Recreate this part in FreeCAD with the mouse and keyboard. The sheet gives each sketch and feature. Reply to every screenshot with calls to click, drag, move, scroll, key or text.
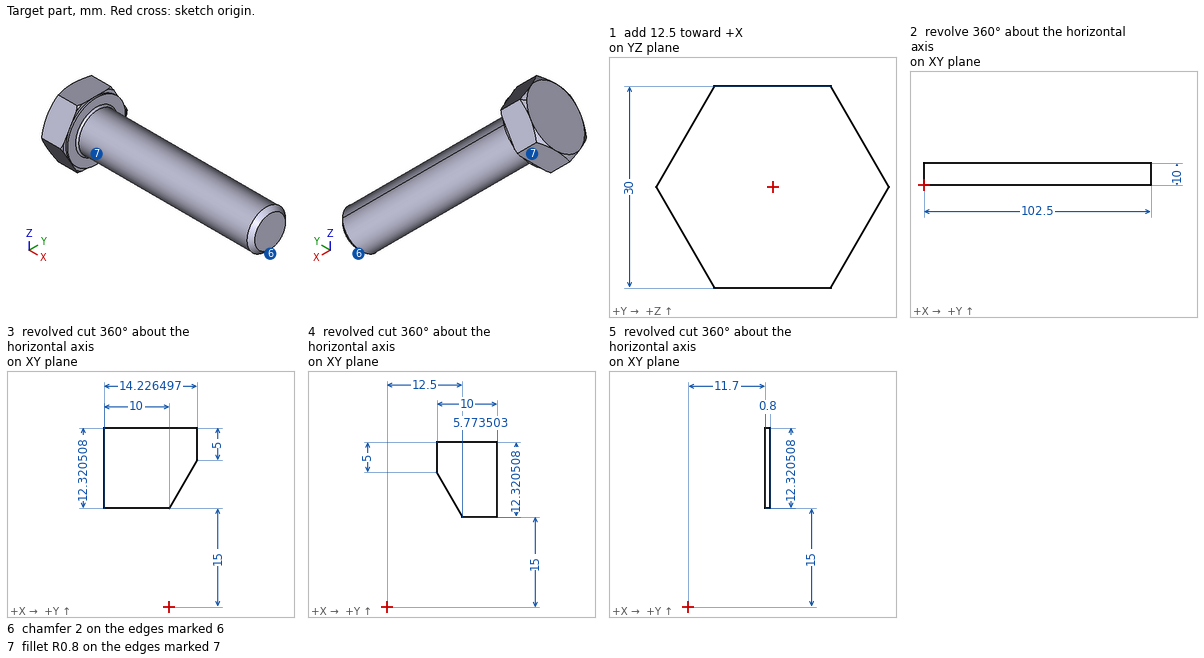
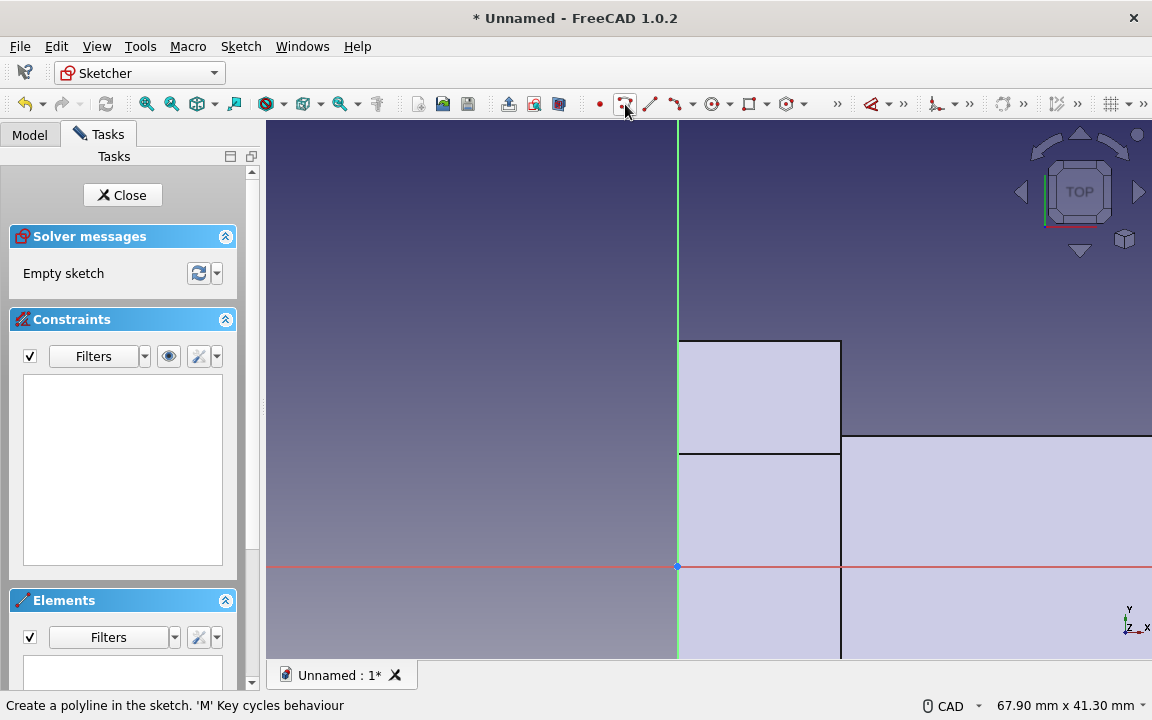
click(678, 371)
click(733, 276)
click(733, 210)
click(547, 210)
click(547, 371)
click(678, 372)
key(Escape)
key(Escape)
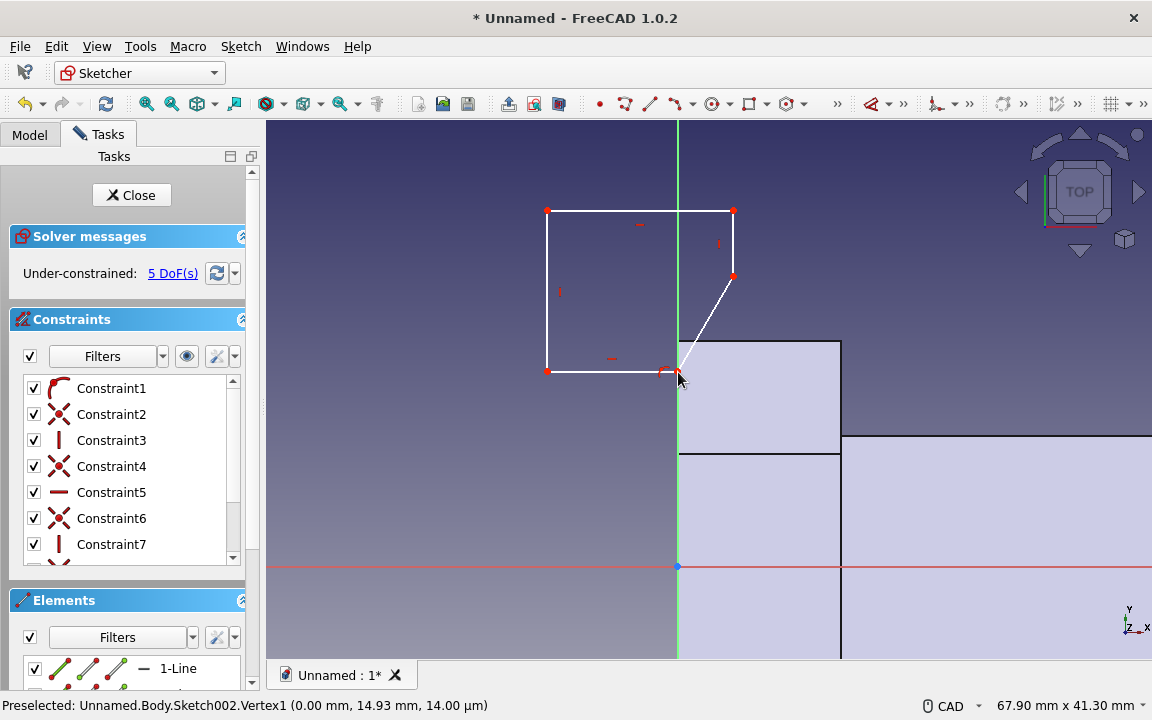
click(733, 257)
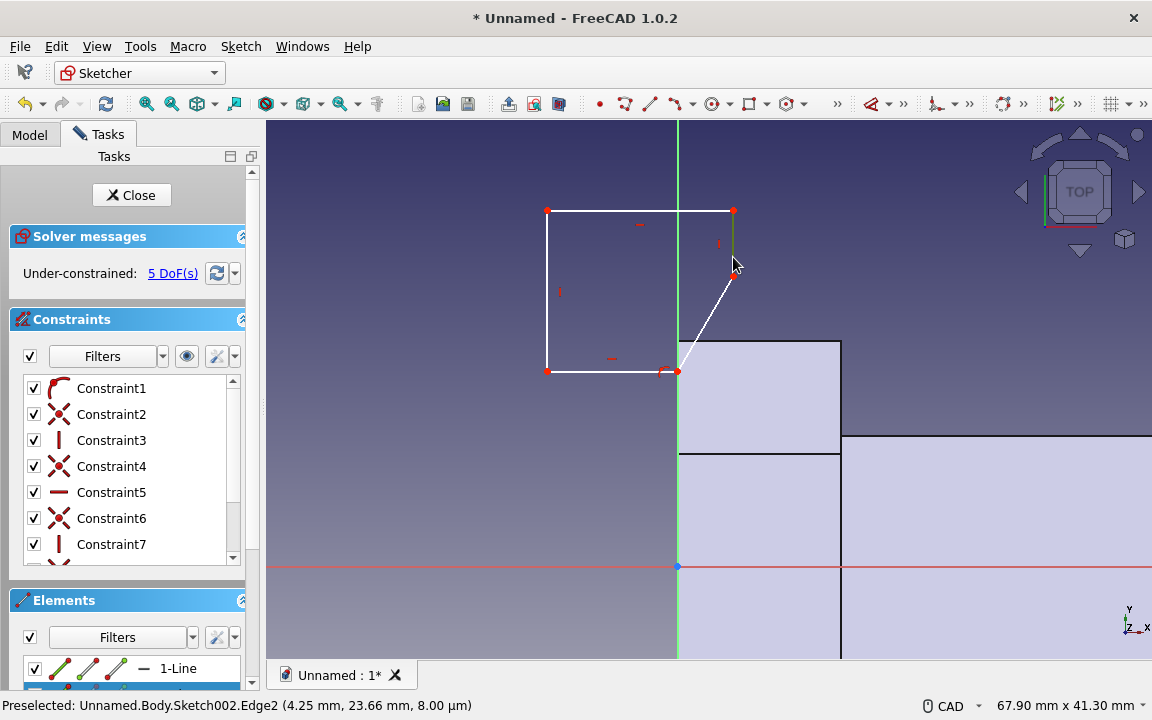
key(i)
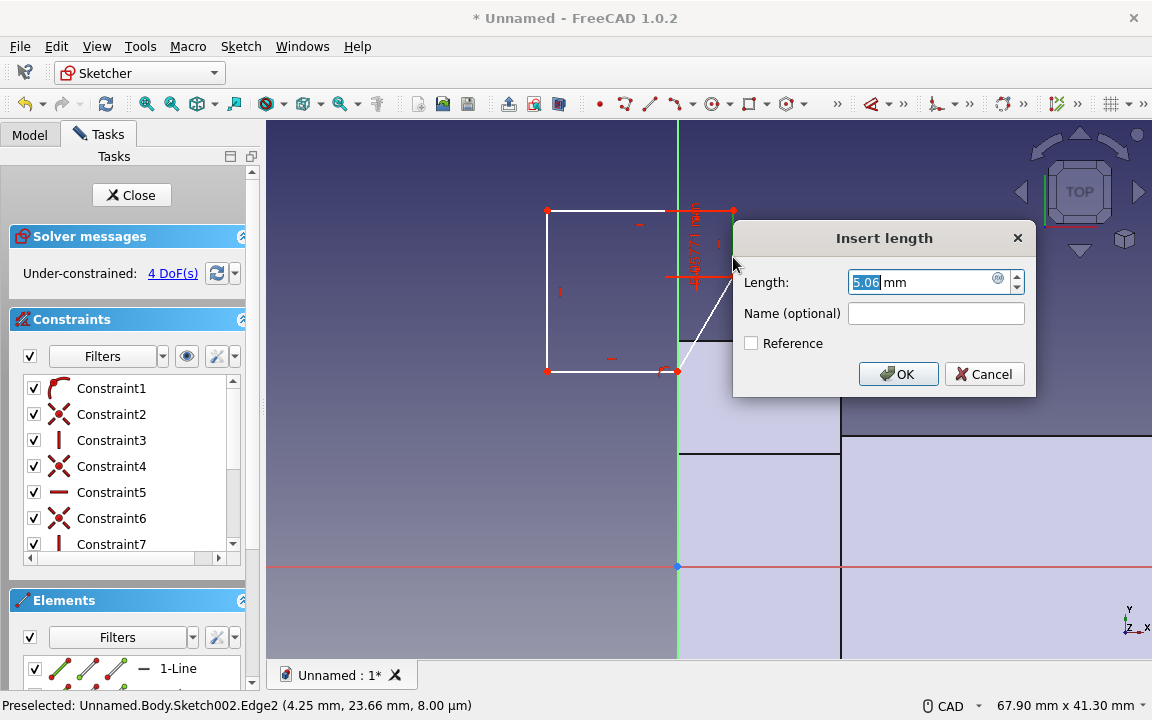
text(5)
key(Return)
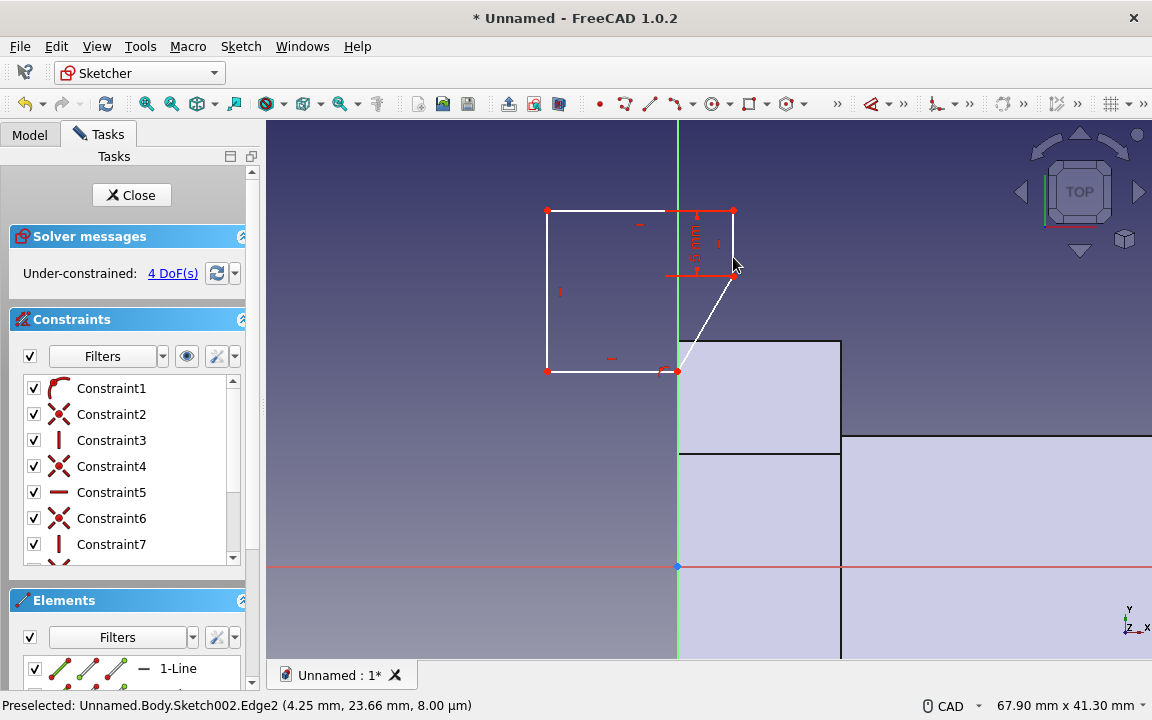
click(586, 372)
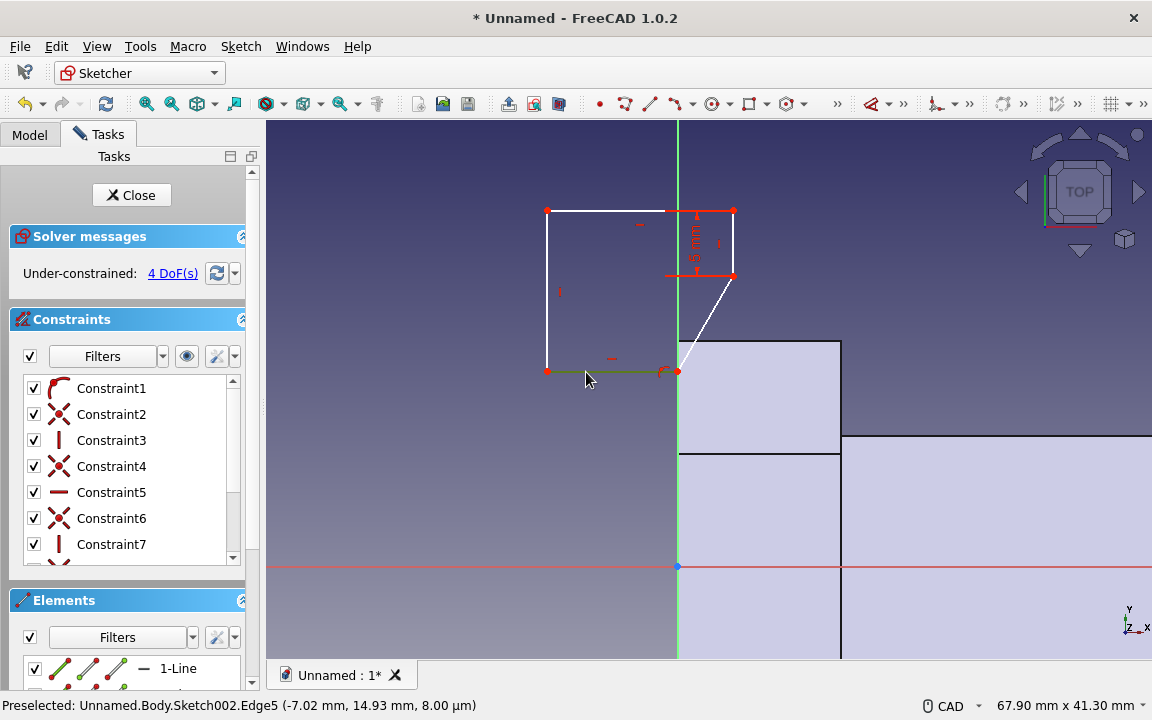
key(l)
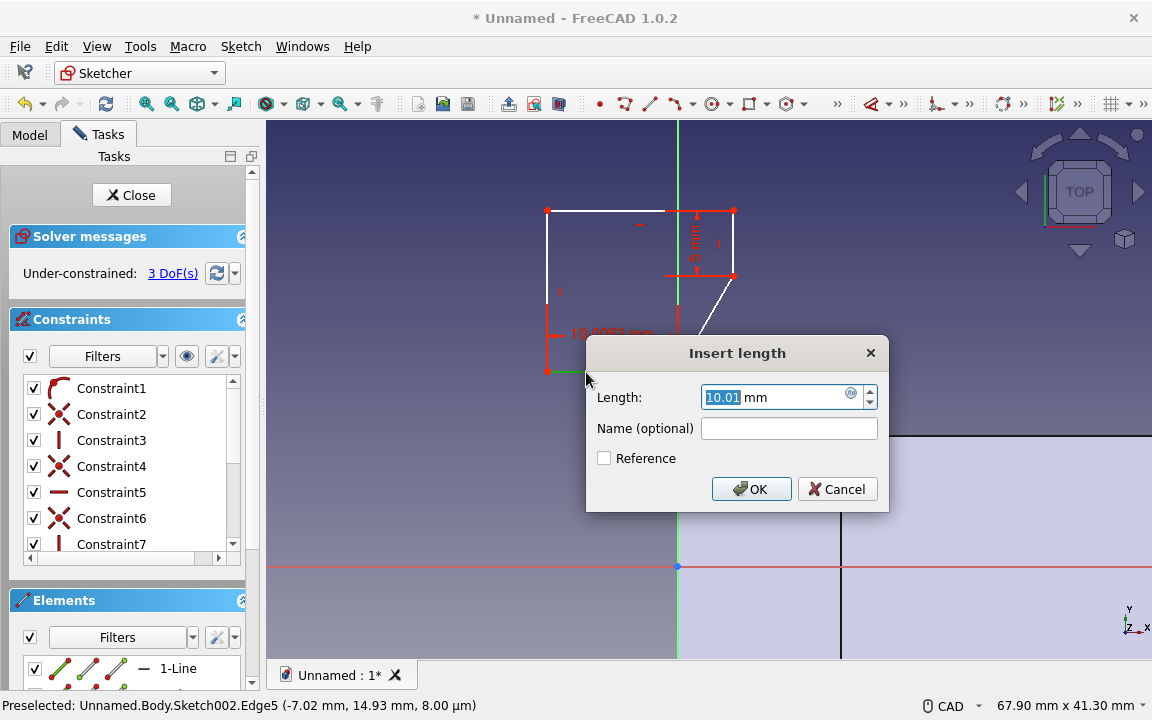
text(10)
key(Return)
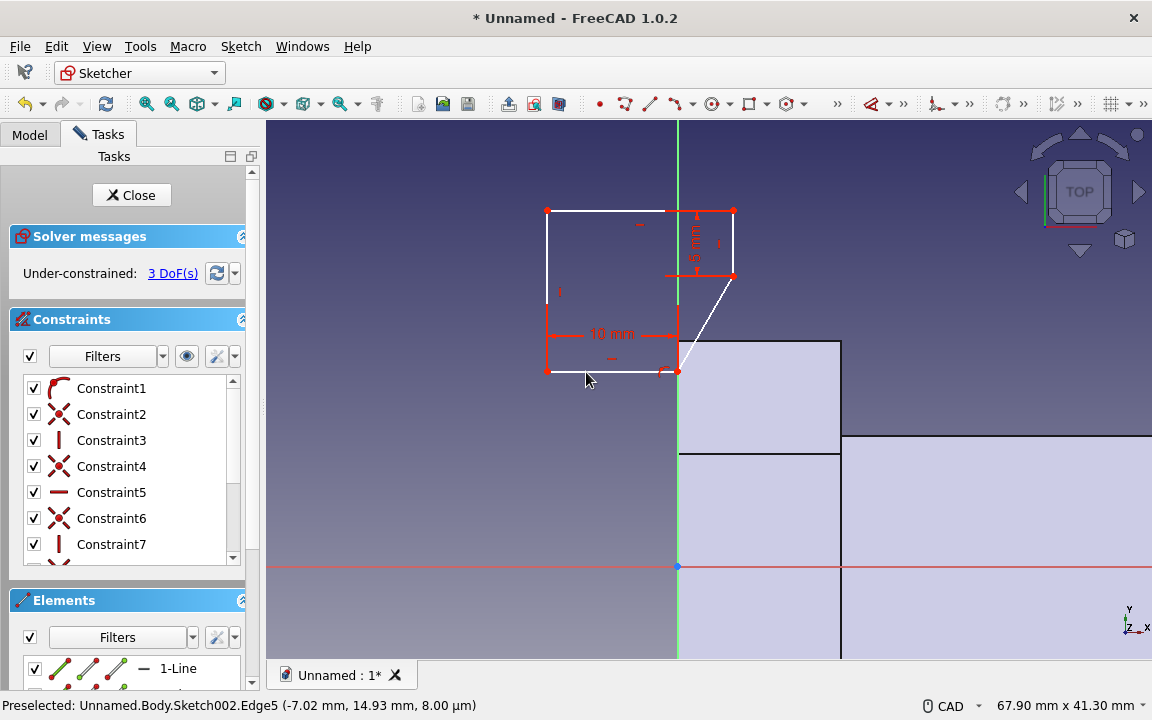
click(678, 372)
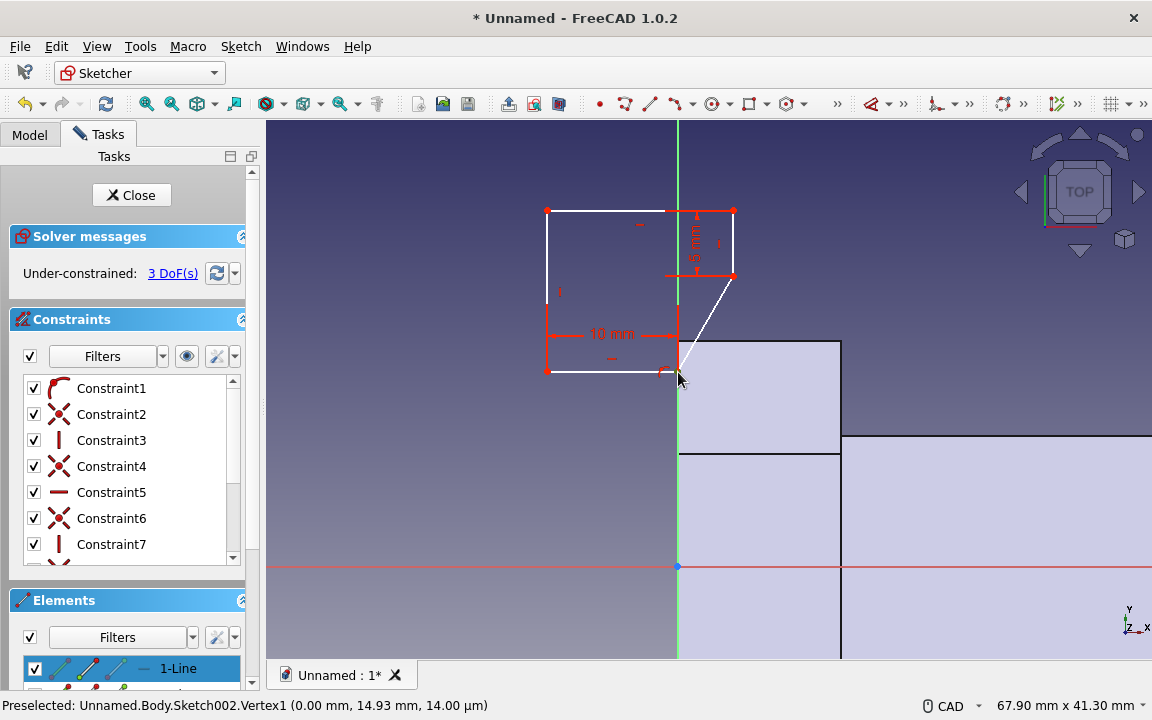
key(i)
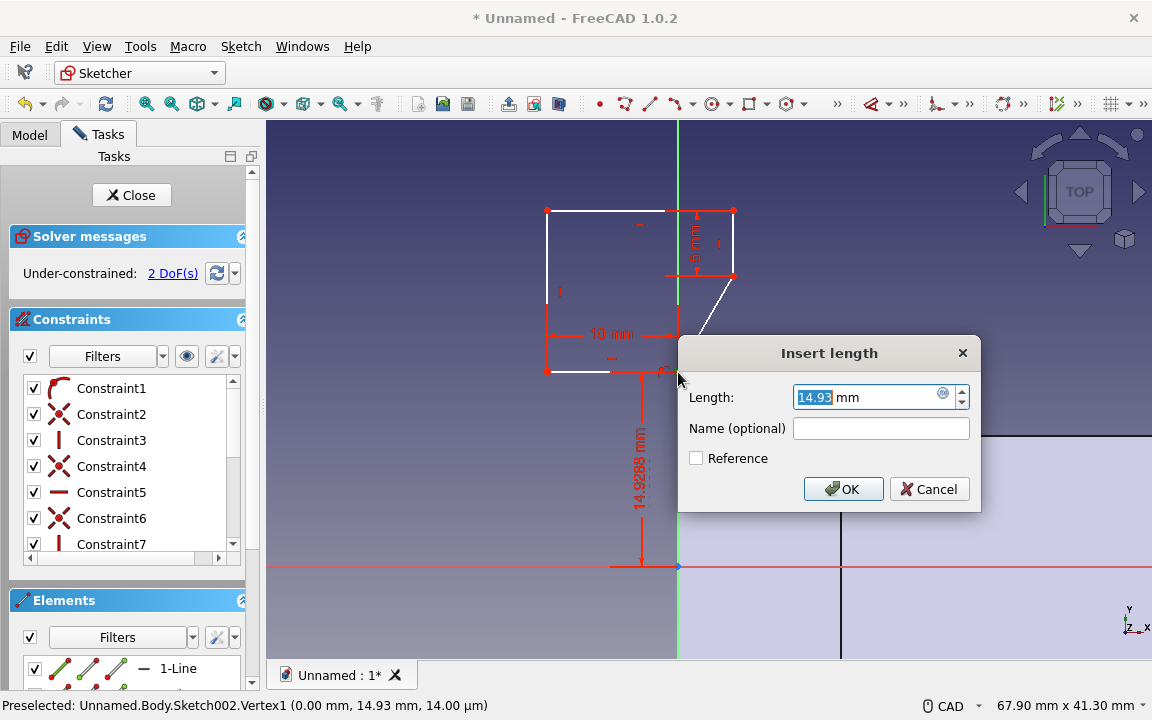
text(15)
key(Return)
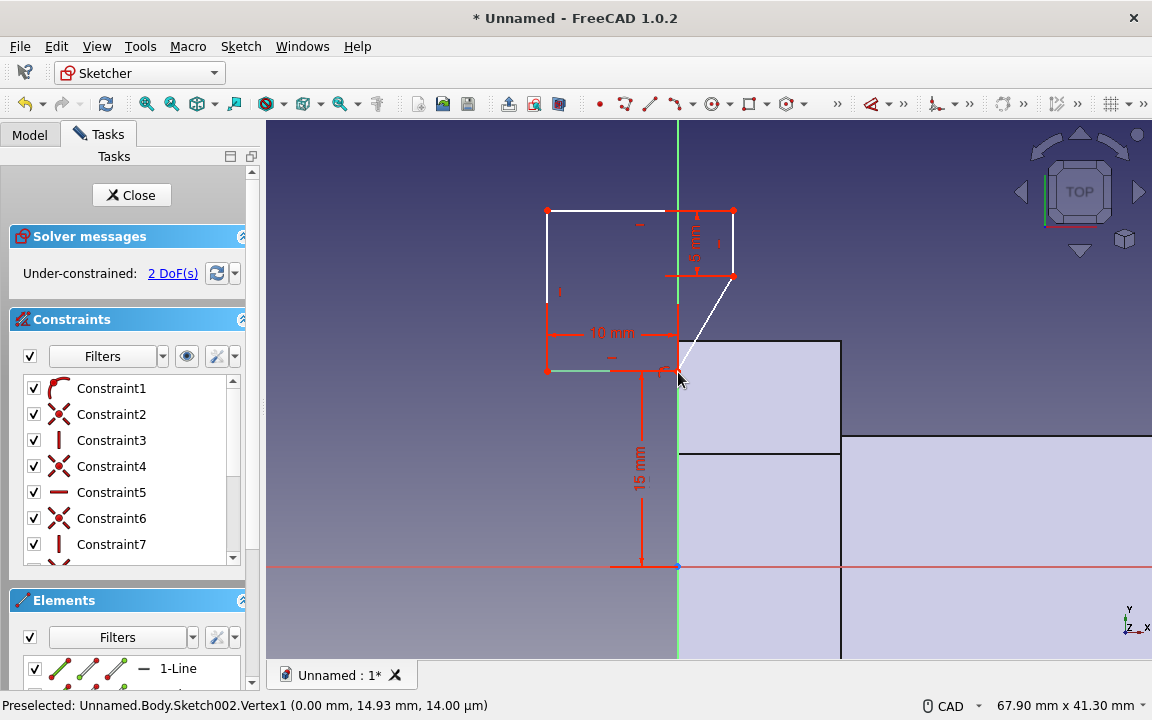
click(677, 211)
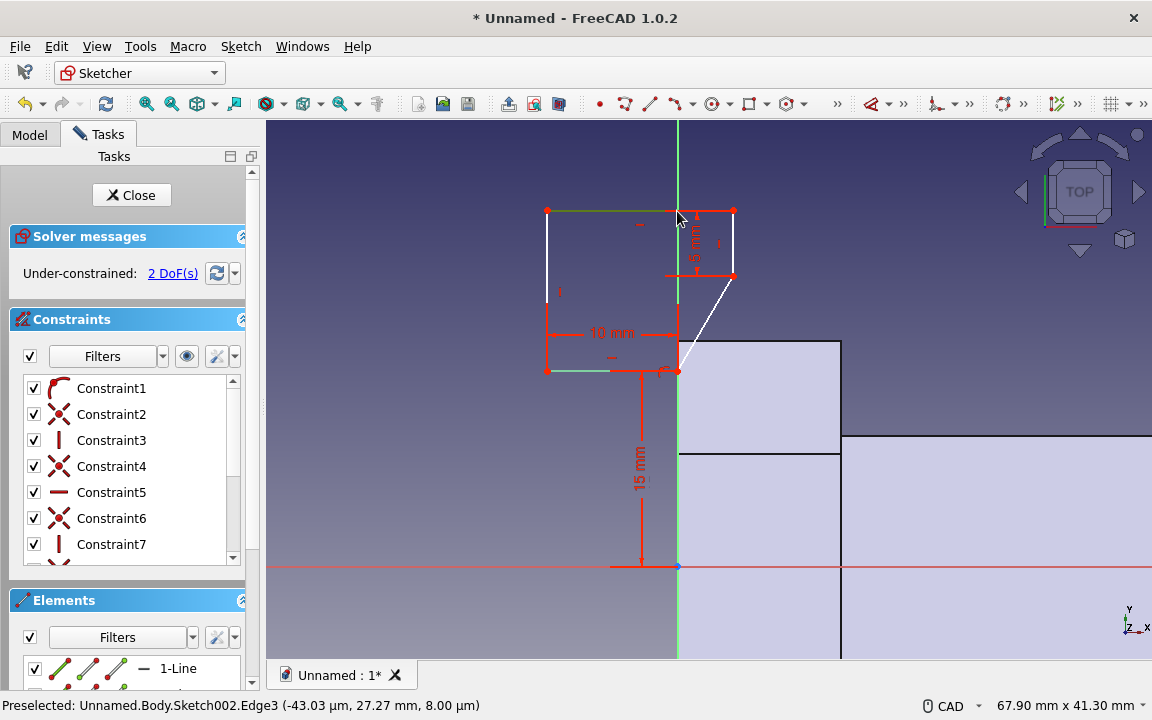
key(l)